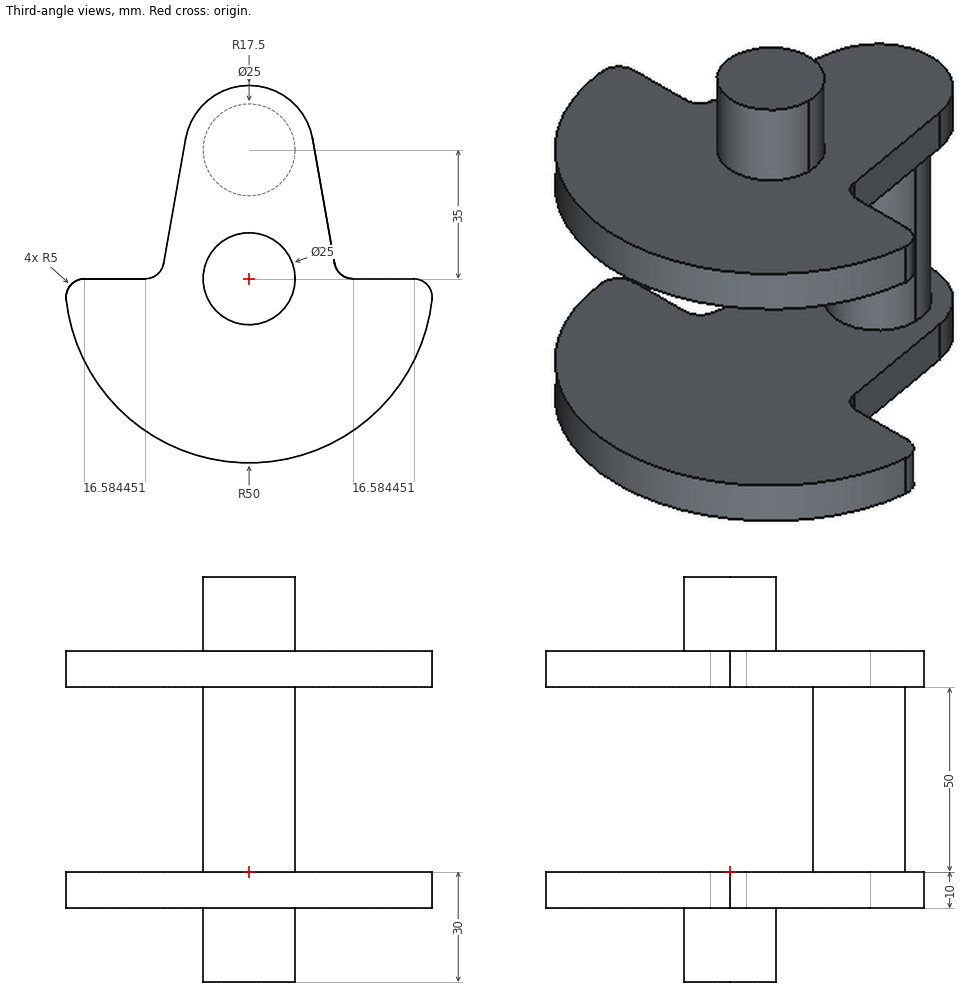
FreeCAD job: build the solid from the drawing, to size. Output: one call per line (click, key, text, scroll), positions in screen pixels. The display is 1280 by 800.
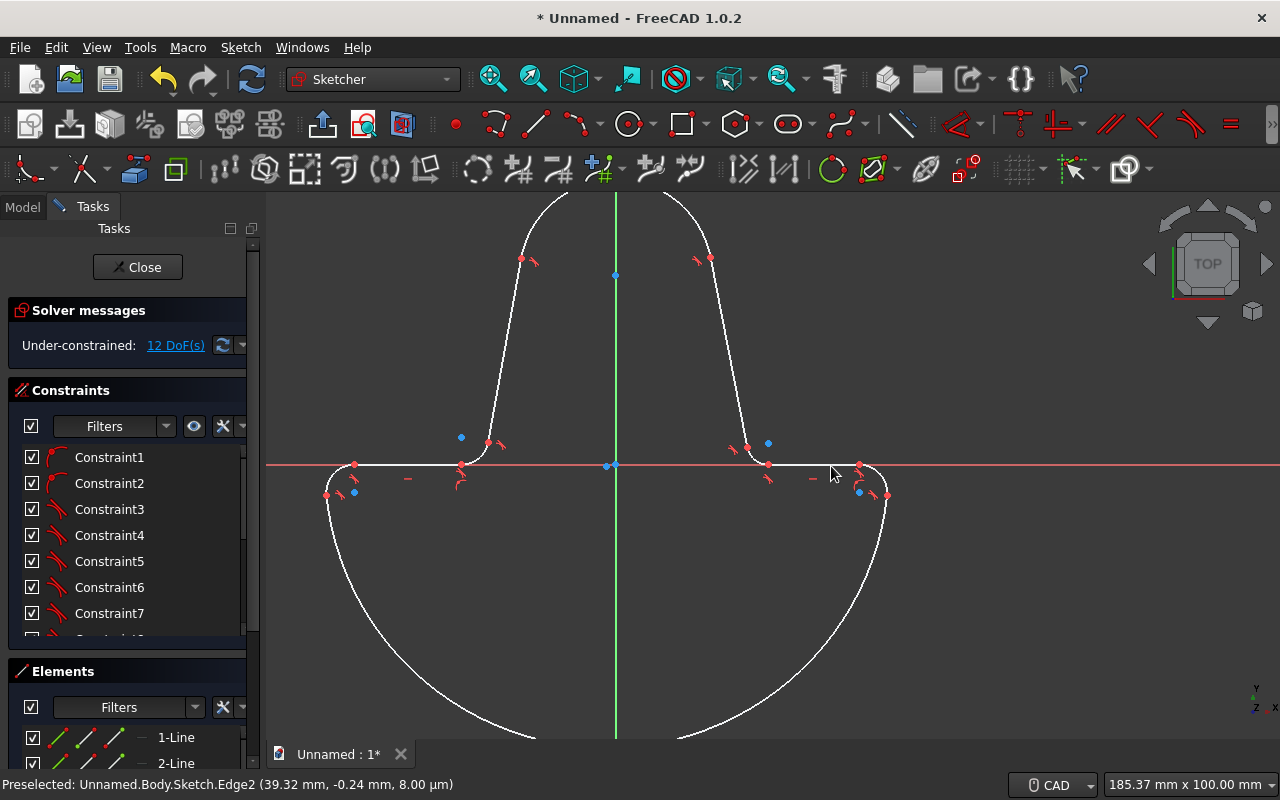
scroll(611, 465, up, 4)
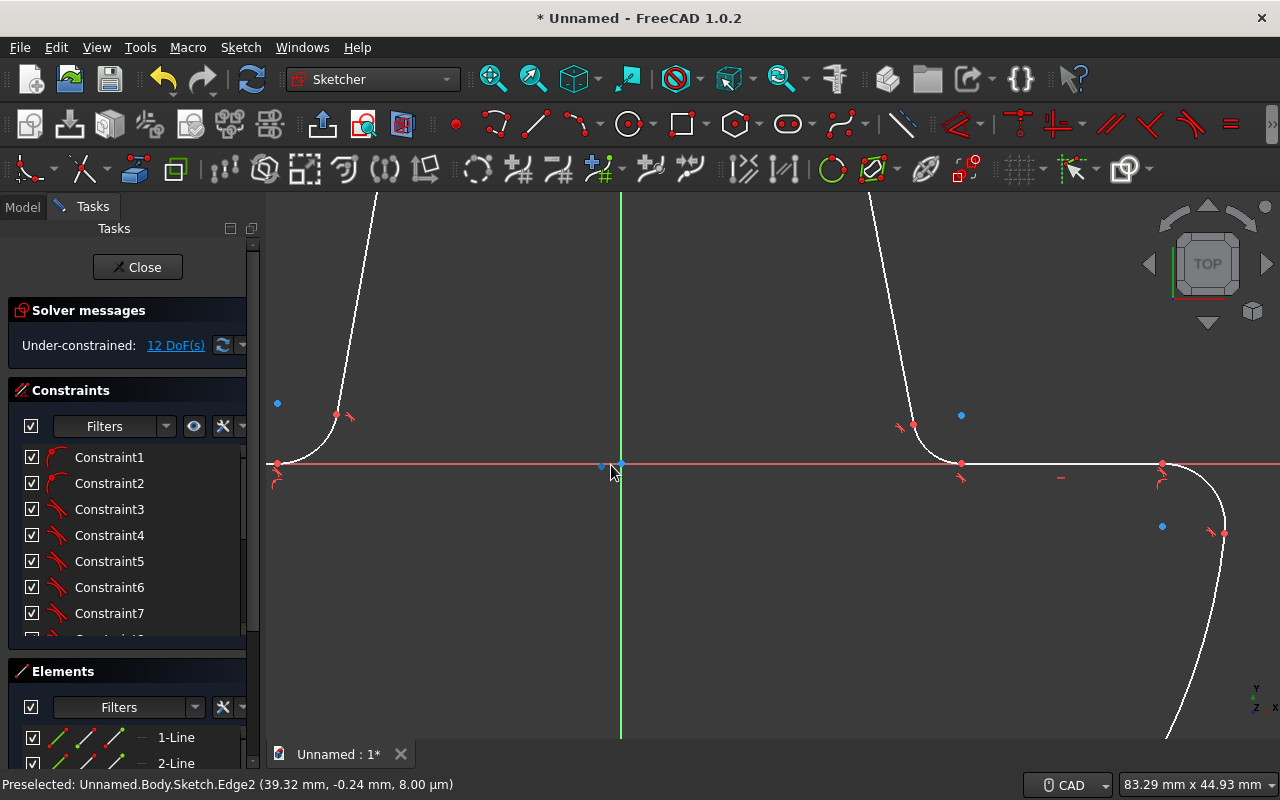
drag(591, 454, 631, 477)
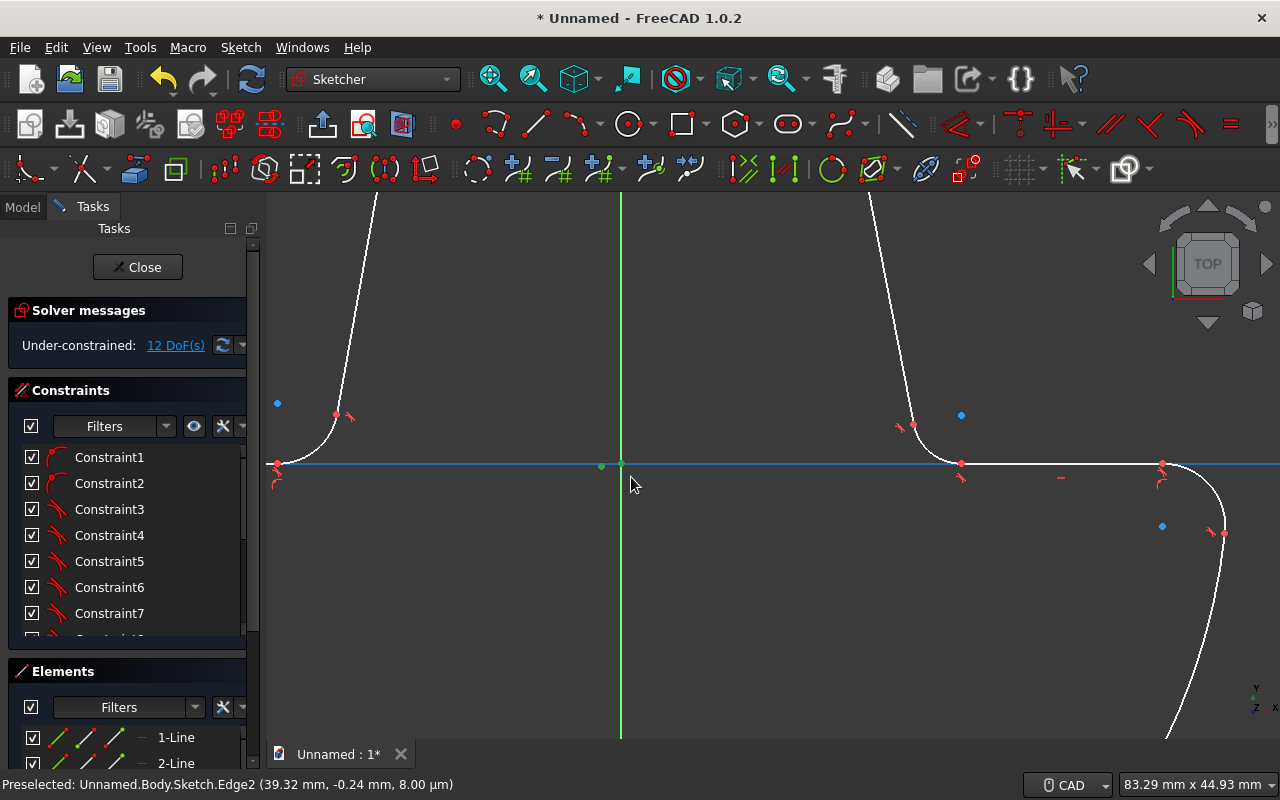
key(c)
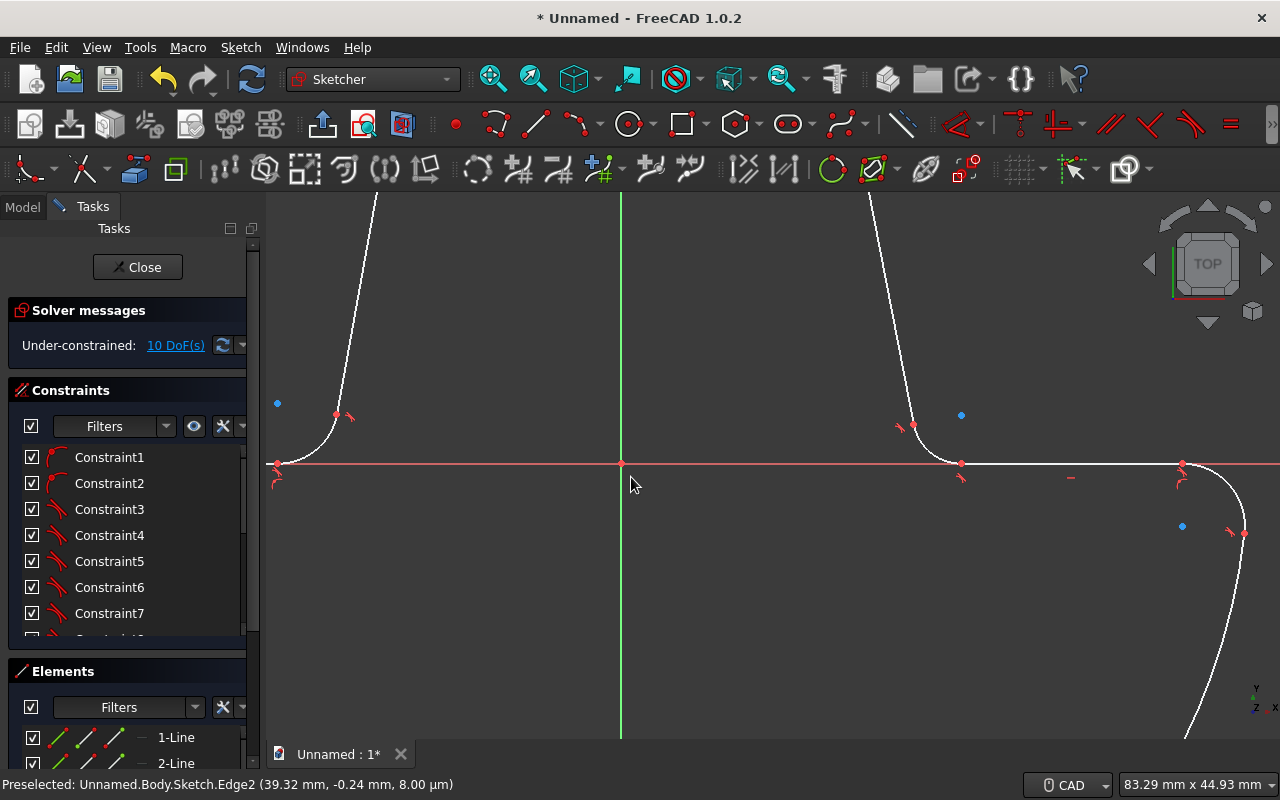
scroll(740, 473, down, 6)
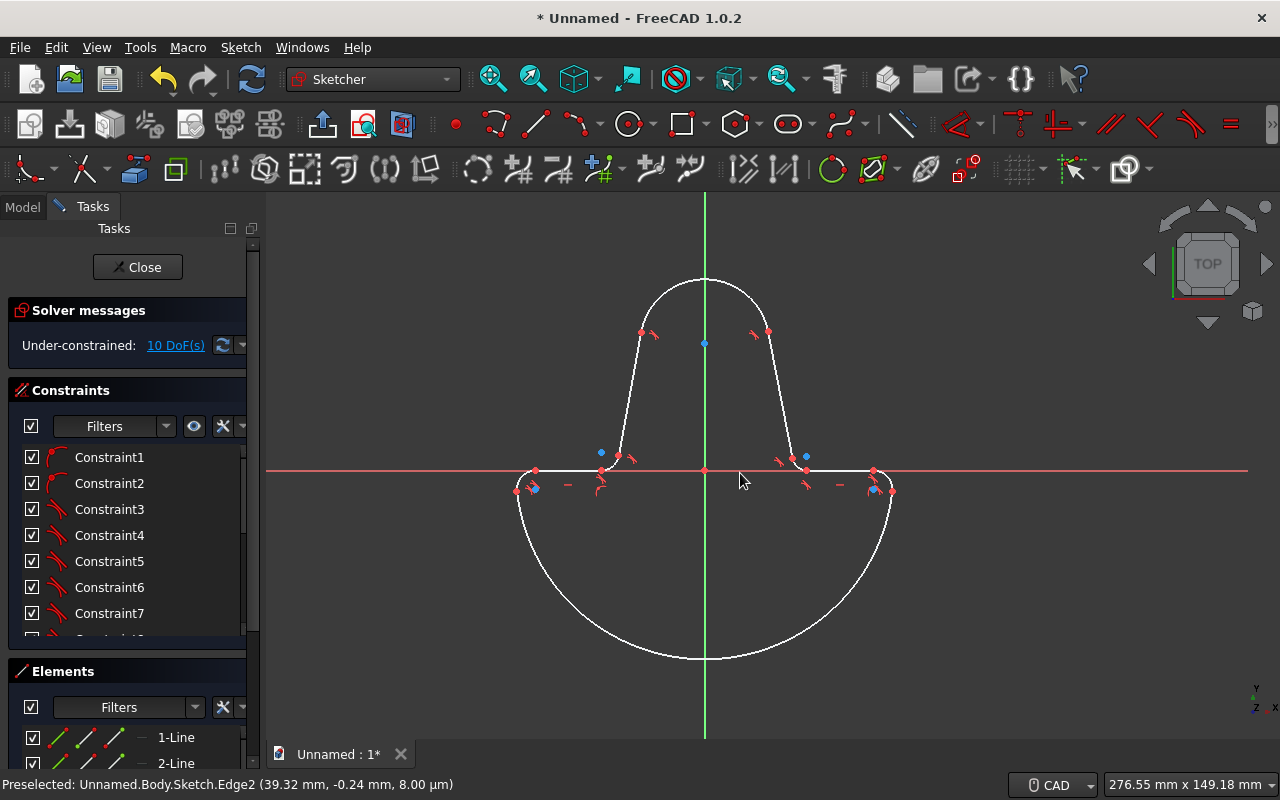
scroll(518, 482, up, 2)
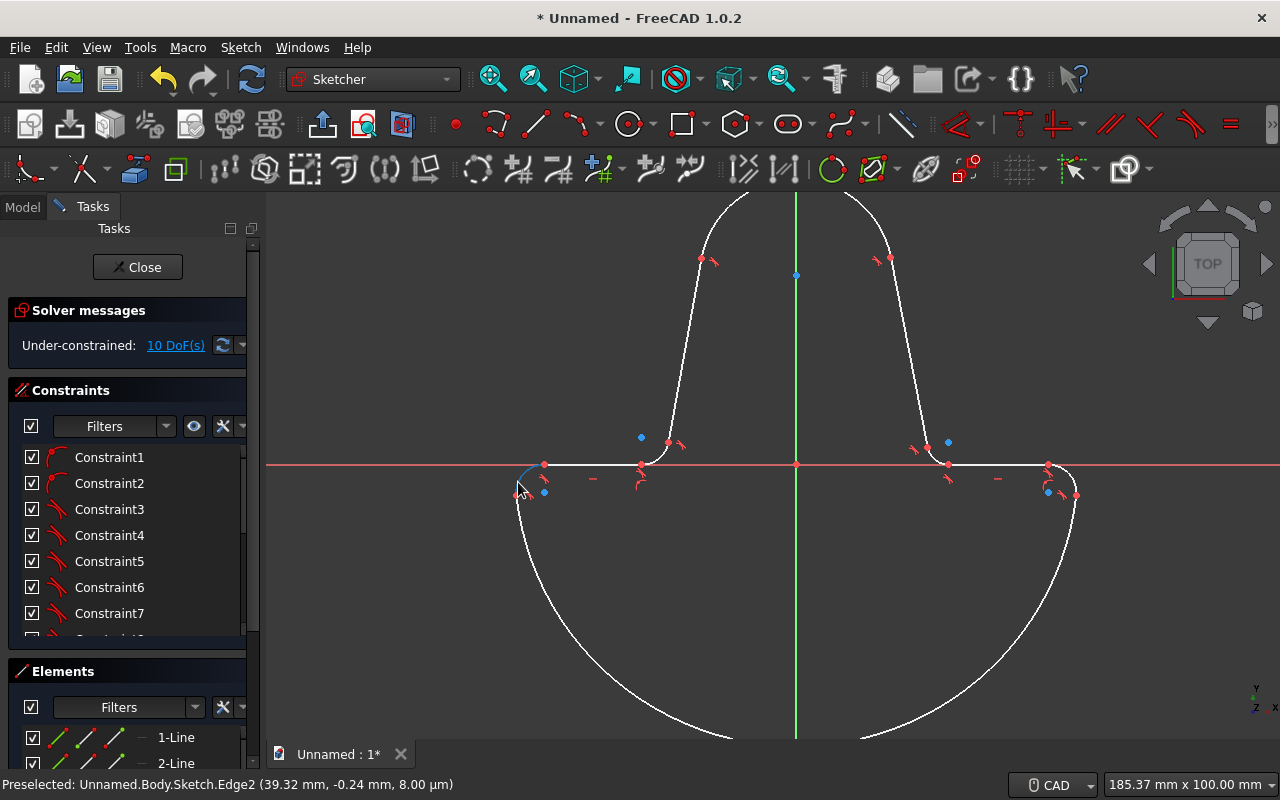
click(518, 482)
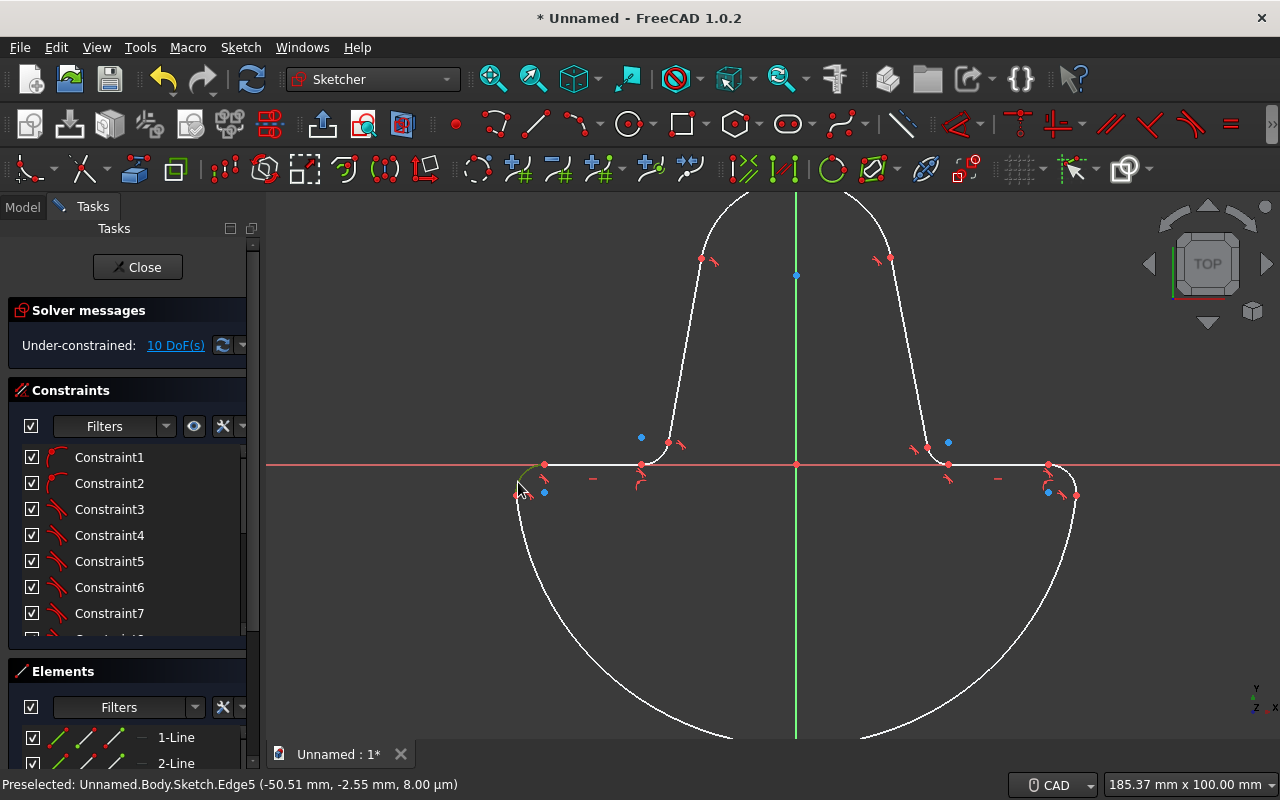
click(1074, 482)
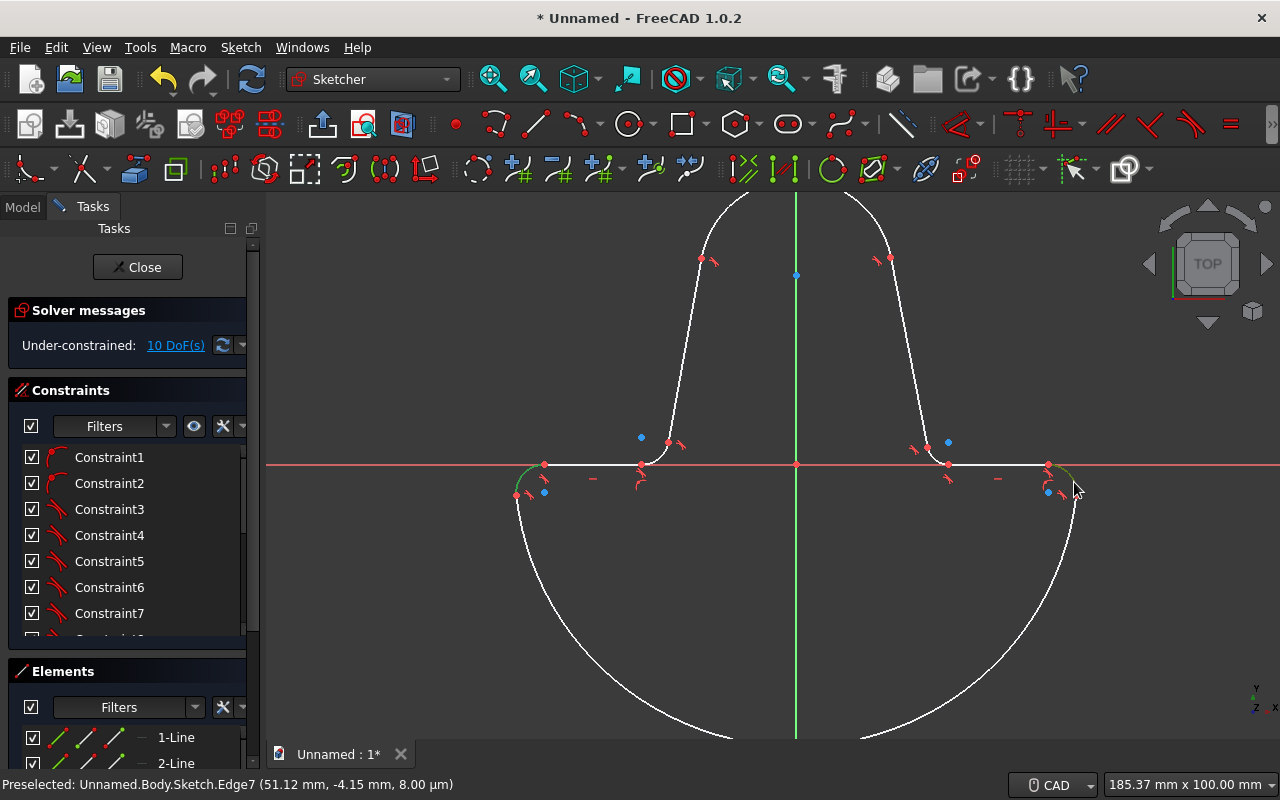
scroll(940, 463, up, 3)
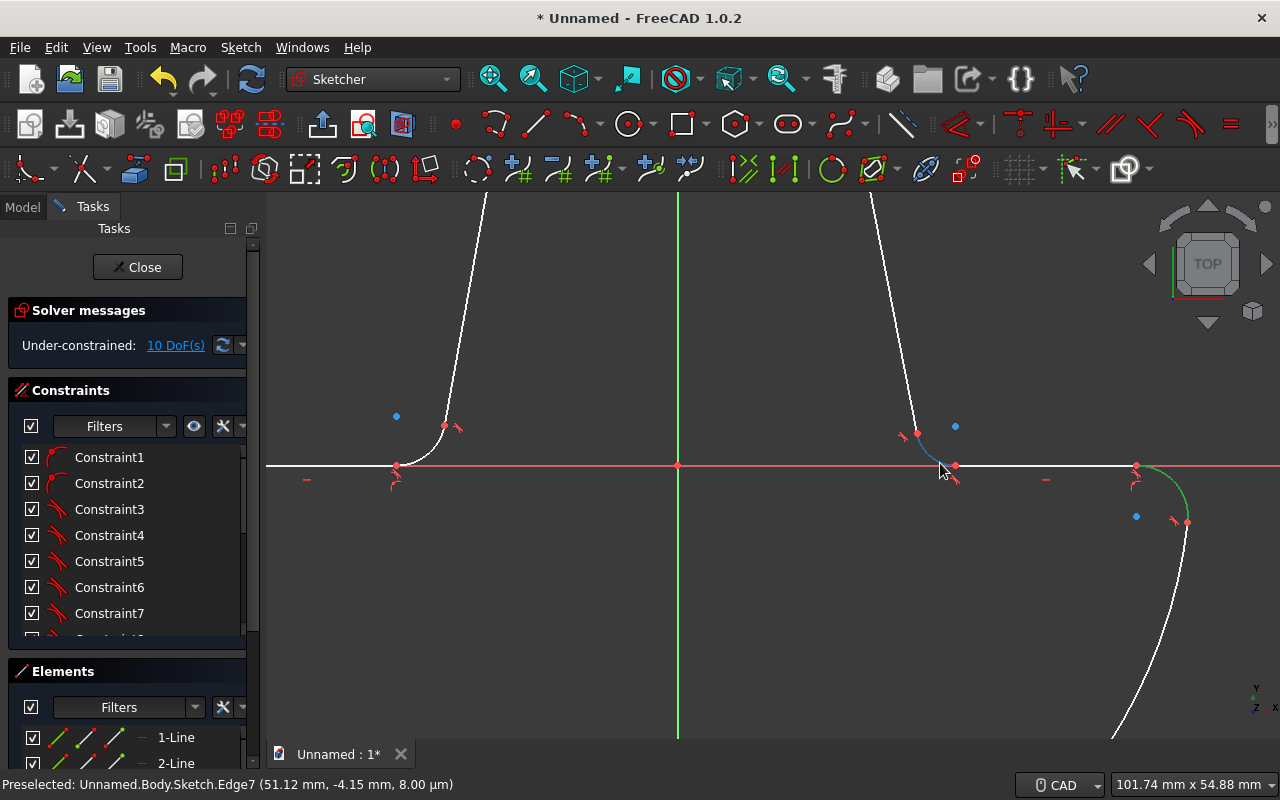
click(940, 462)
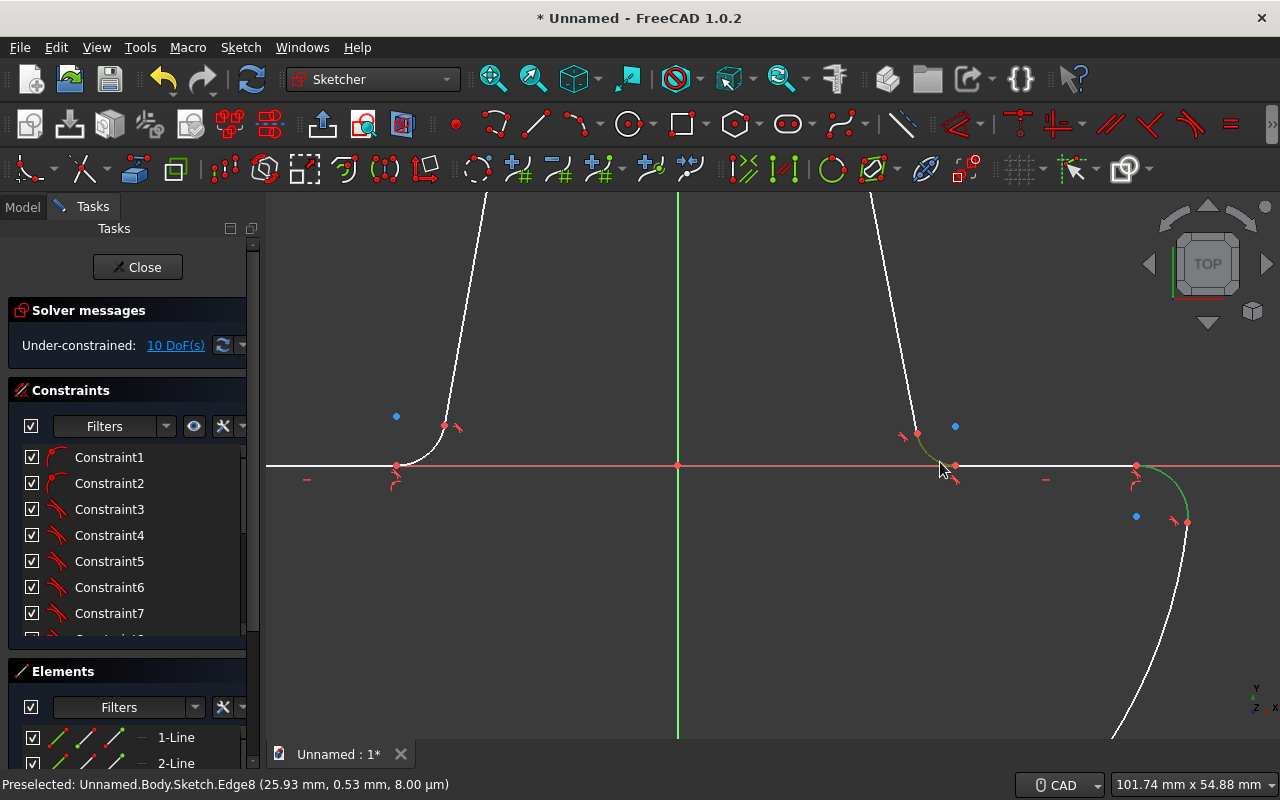
click(437, 444)